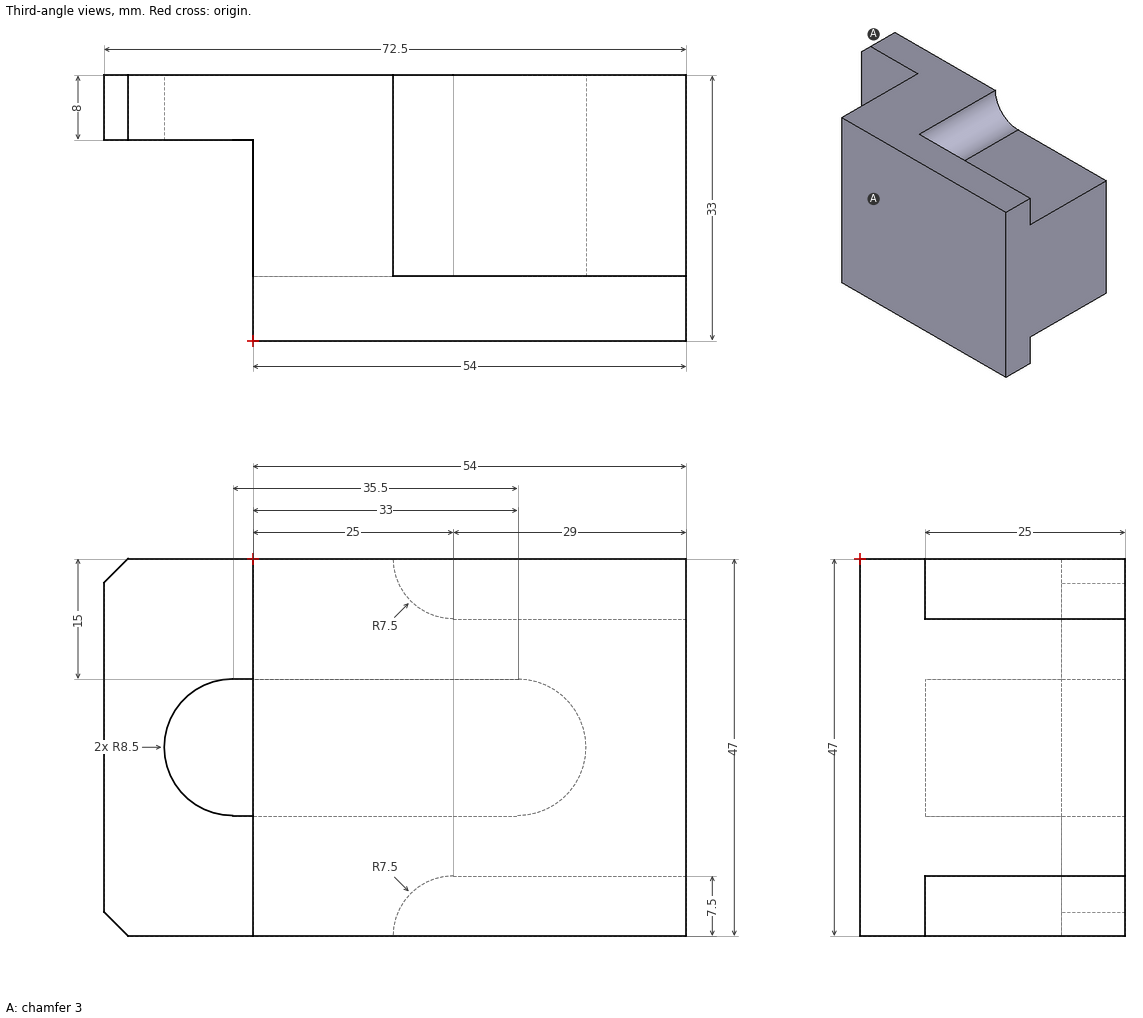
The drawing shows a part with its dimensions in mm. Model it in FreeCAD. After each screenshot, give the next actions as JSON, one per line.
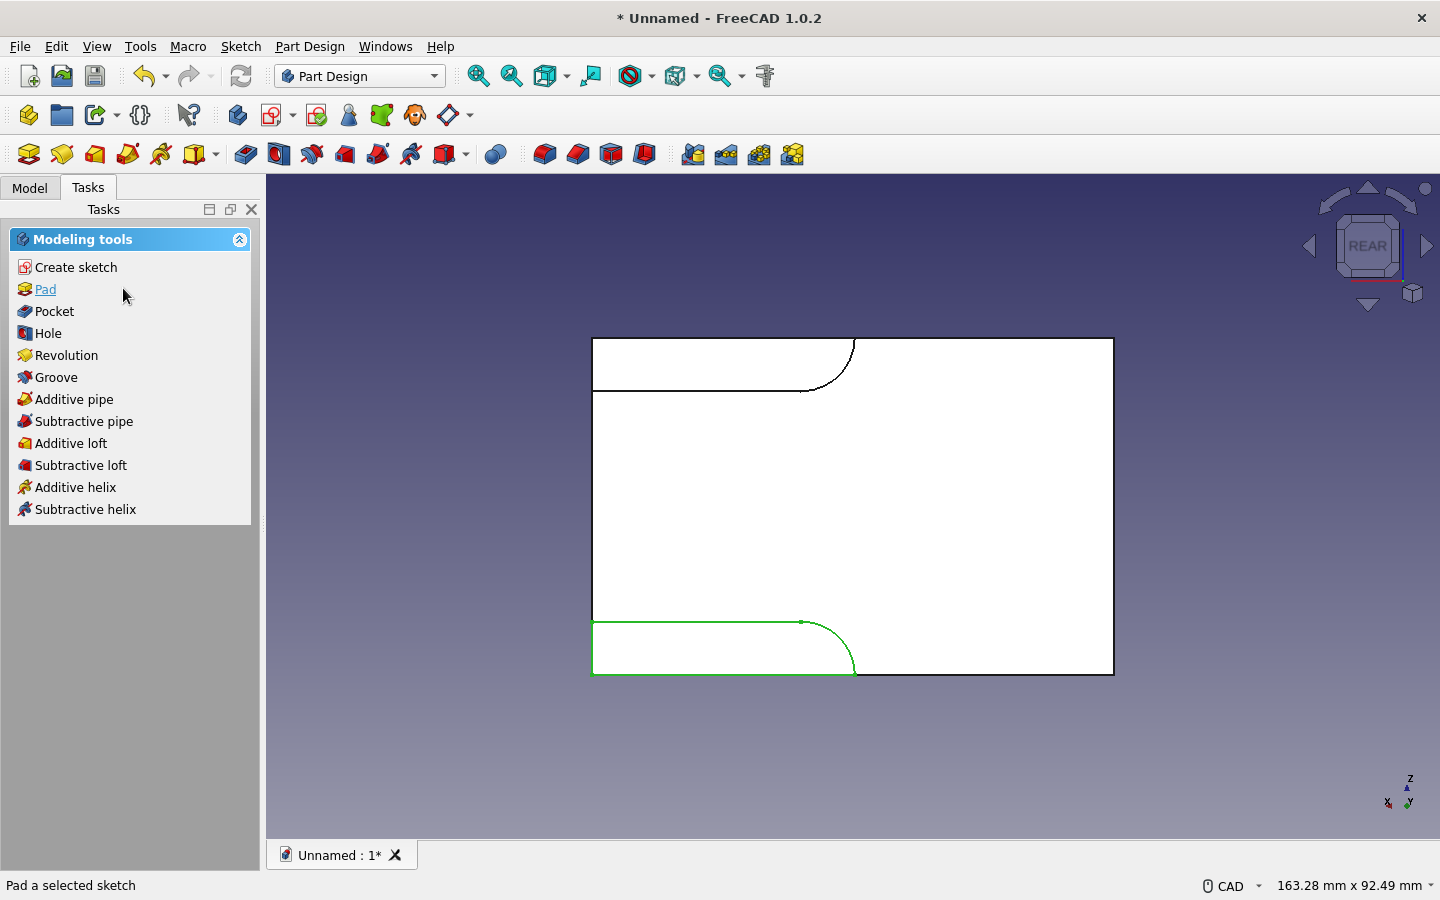
{"action": "left_click", "coordinate": [246, 154]}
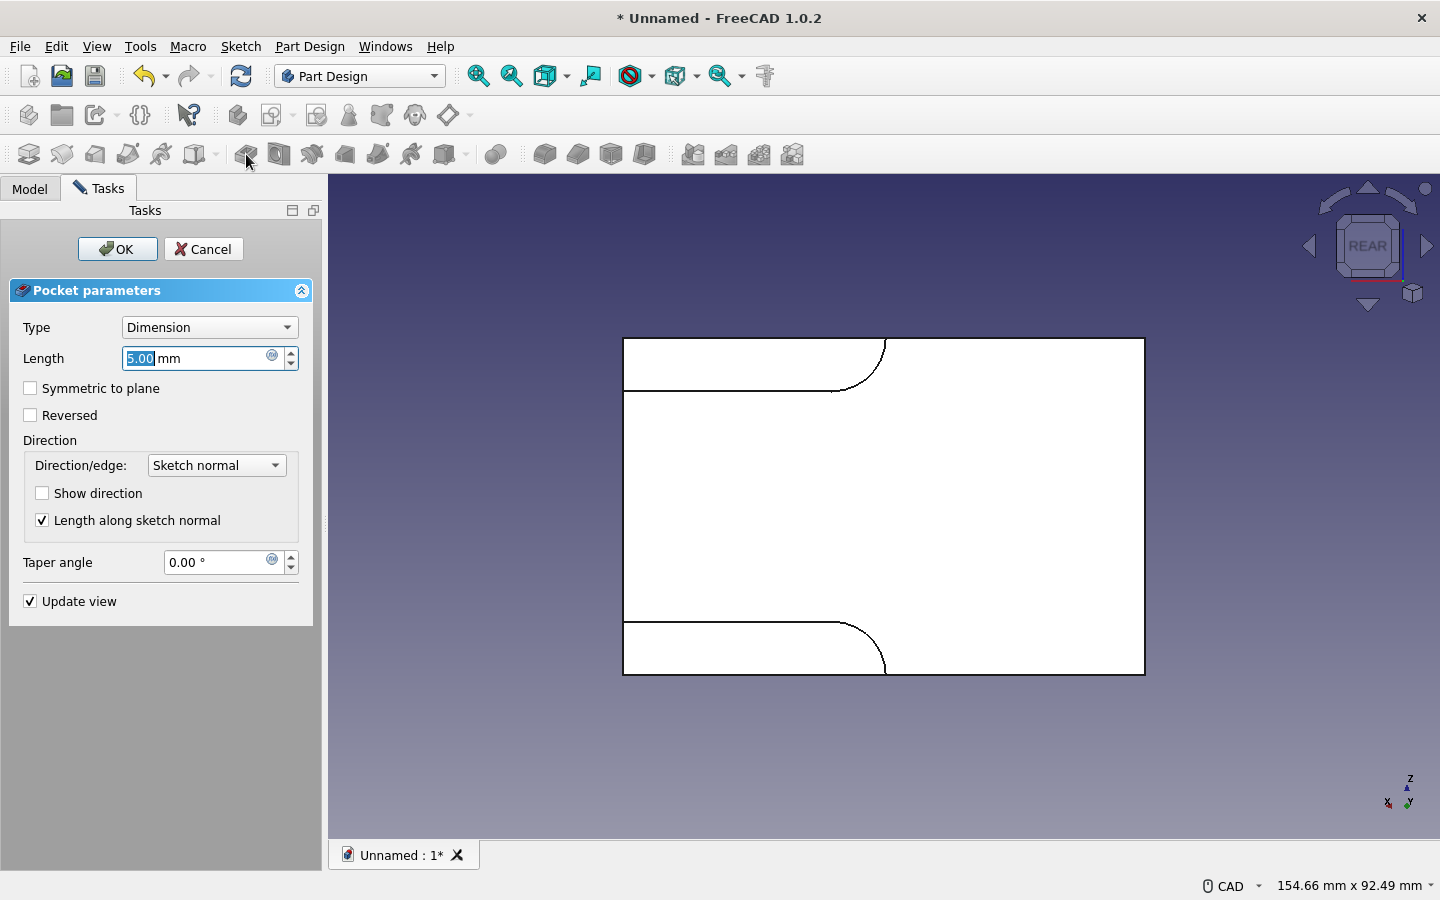
{"action": "type", "text": "25"}
{"action": "key", "text": "Tab"}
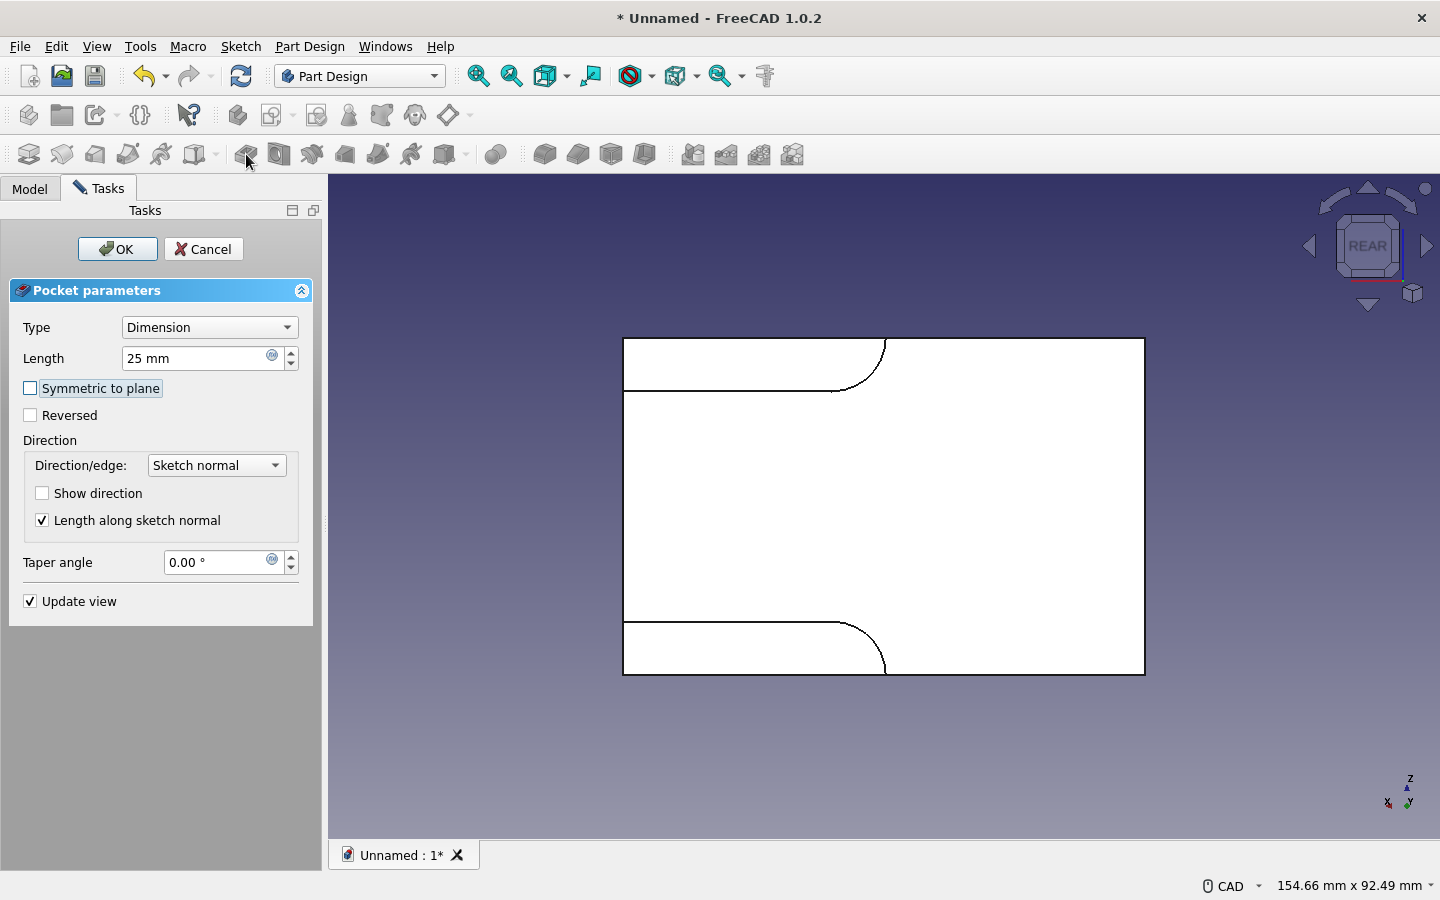
{"action": "left_click", "coordinate": [118, 249]}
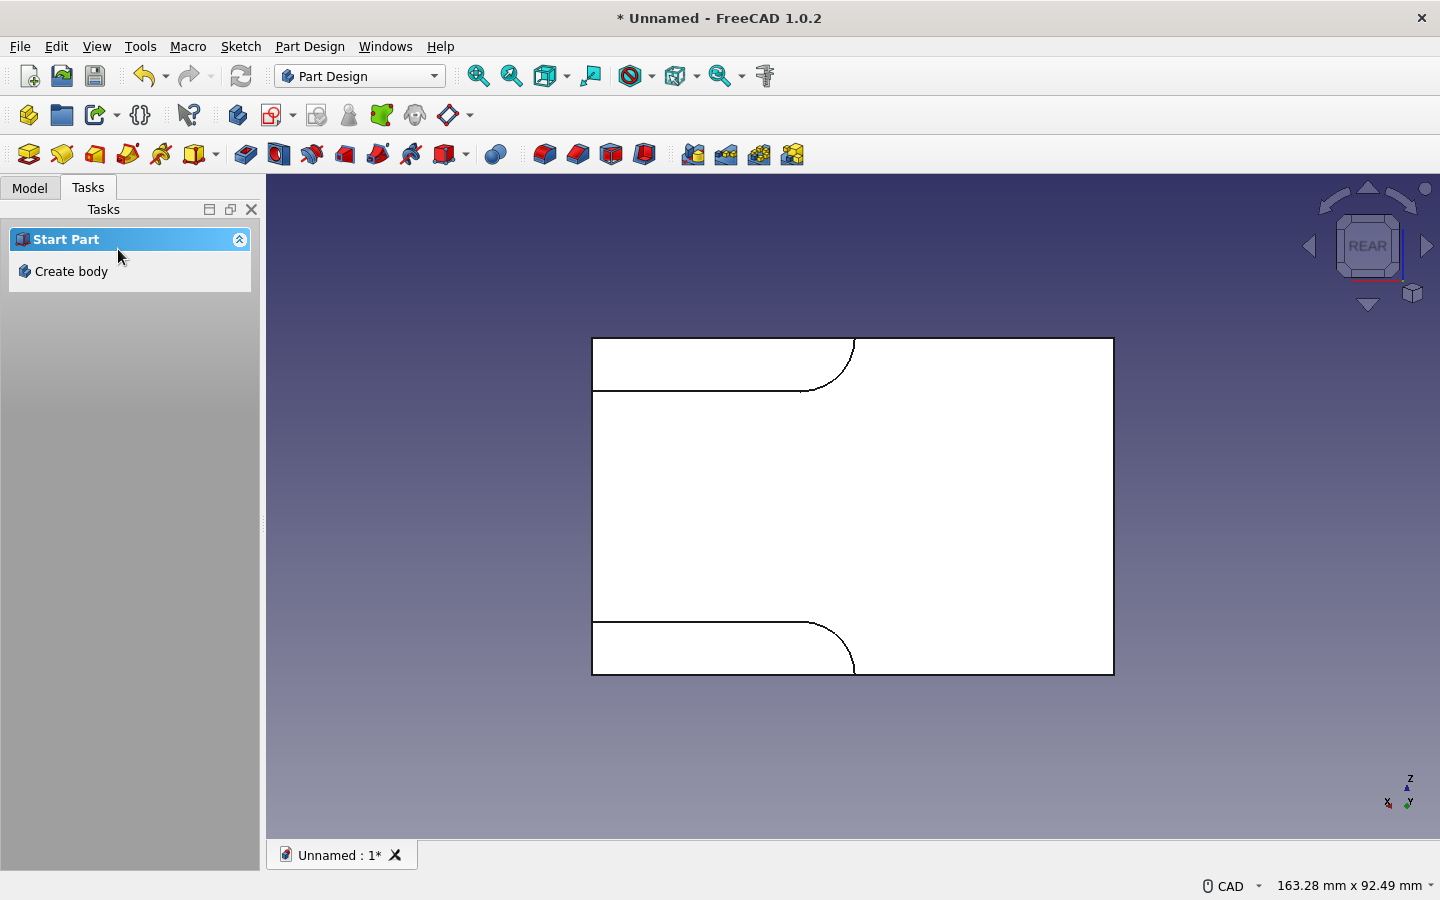
{"action": "left_click", "coordinate": [927, 505]}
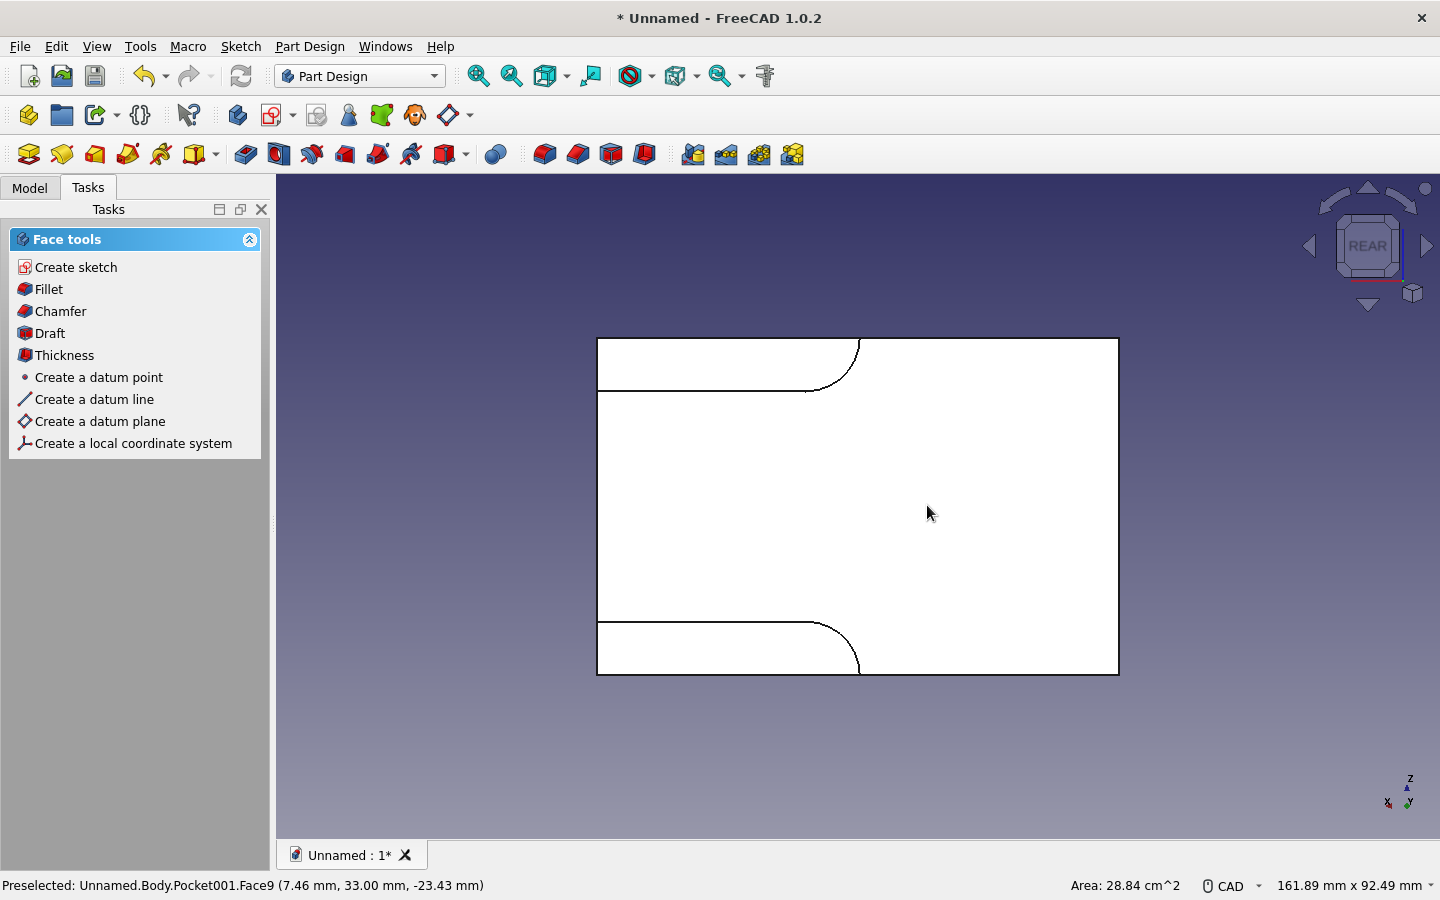
{"action": "left_click", "coordinate": [270, 116]}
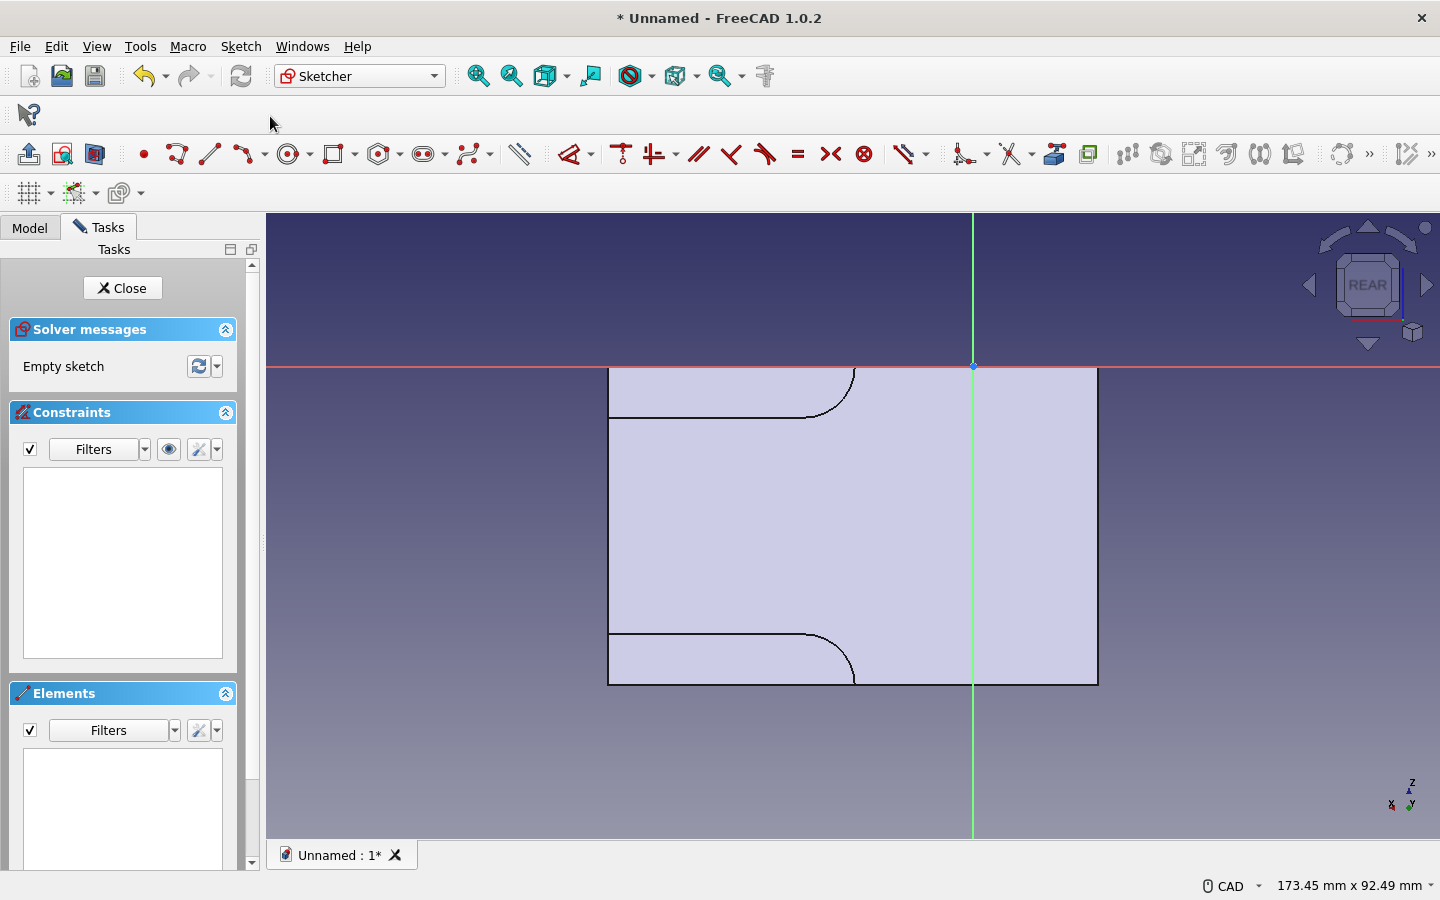
{"action": "scroll", "coordinate": [974, 413], "scroll_direction": "up", "scroll_amount": 3}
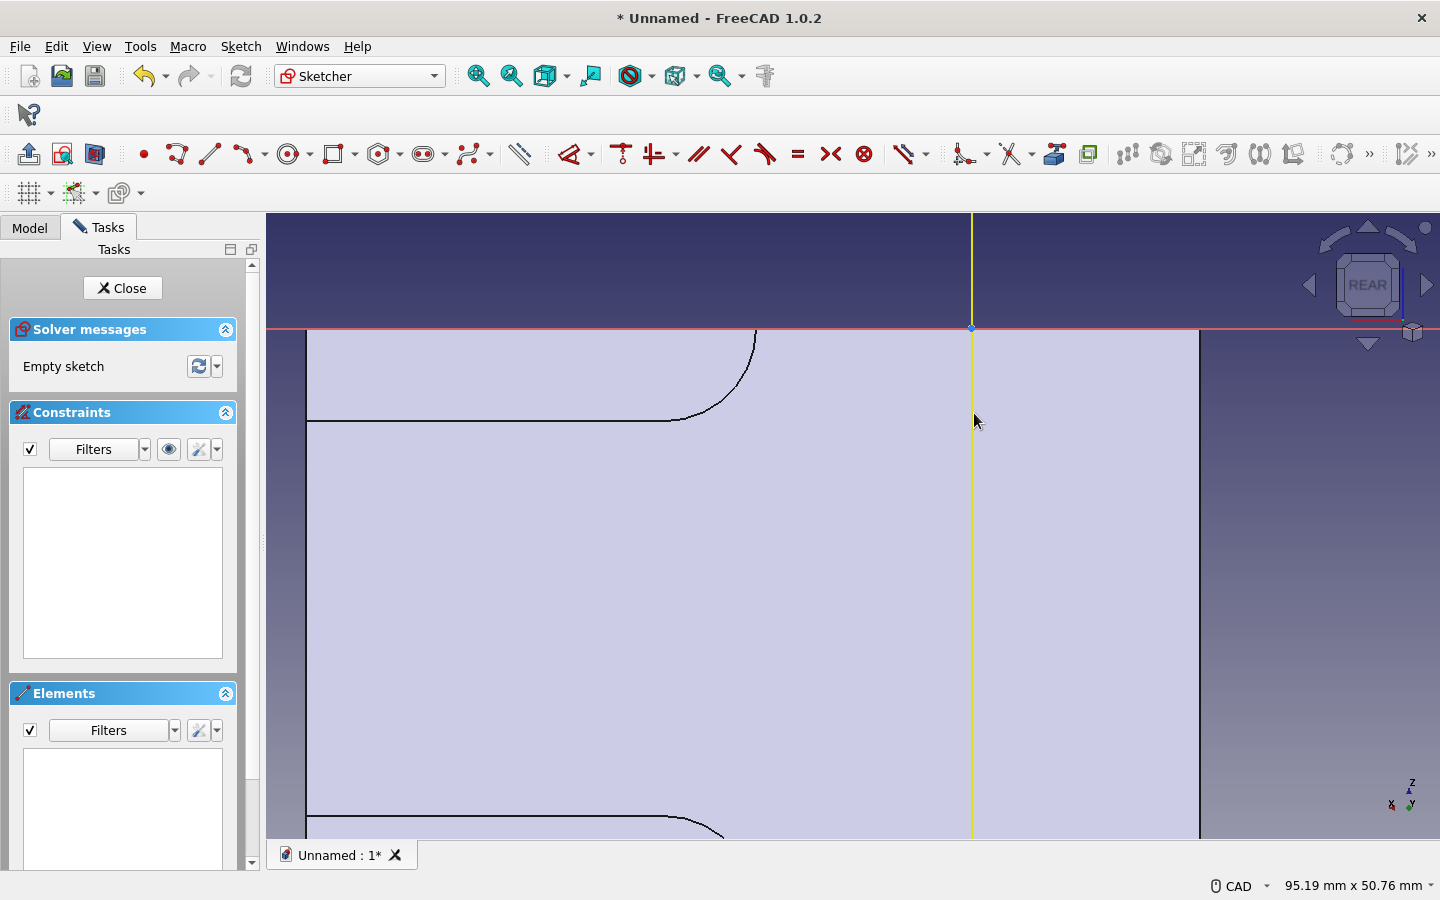
{"action": "left_click", "coordinate": [422, 154]}